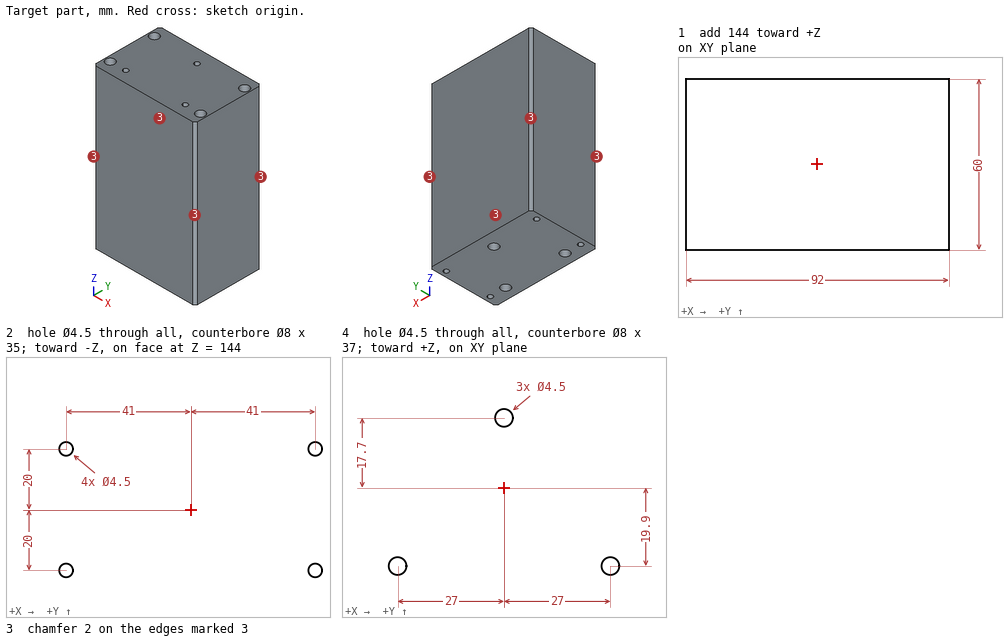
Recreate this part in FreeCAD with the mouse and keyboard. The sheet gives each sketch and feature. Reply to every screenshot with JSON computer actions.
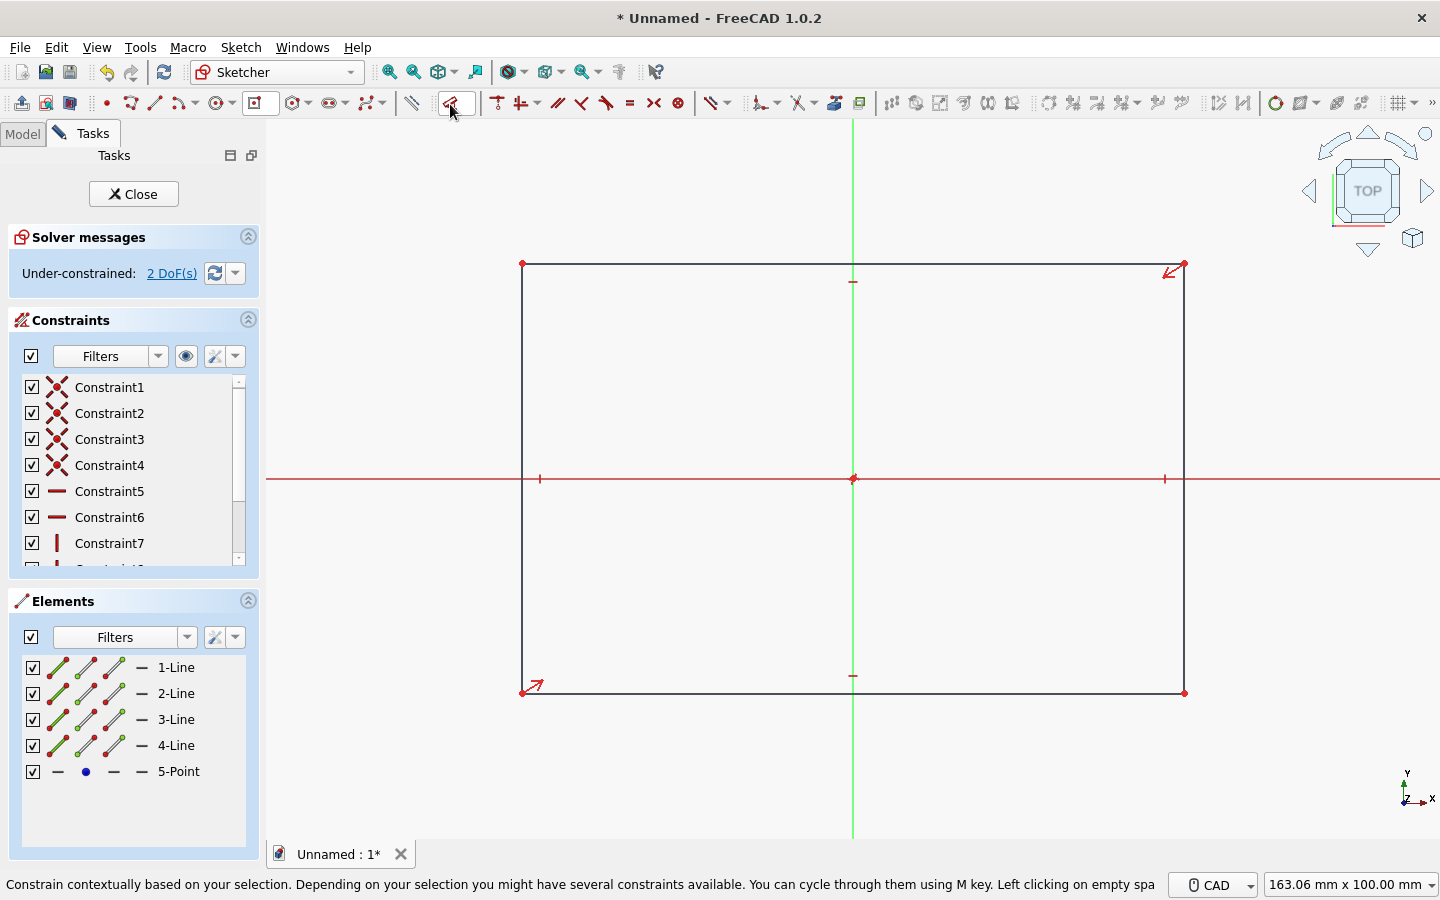
{"action": "left_click", "coordinate": [721, 694]}
{"action": "left_click", "coordinate": [701, 728]}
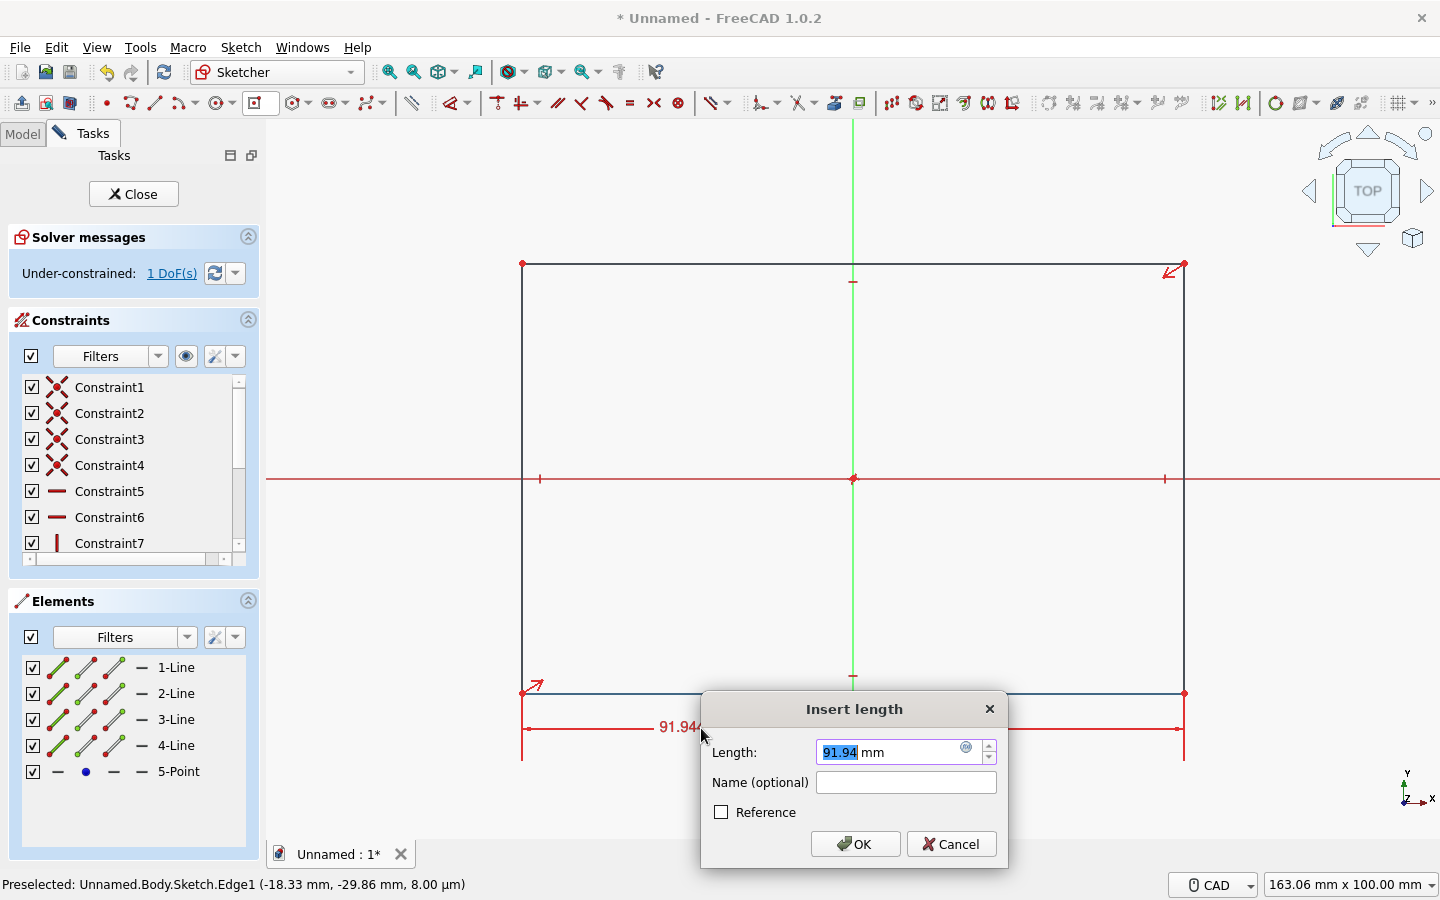
{"action": "type", "text": "92"}
{"action": "key", "text": "Return"}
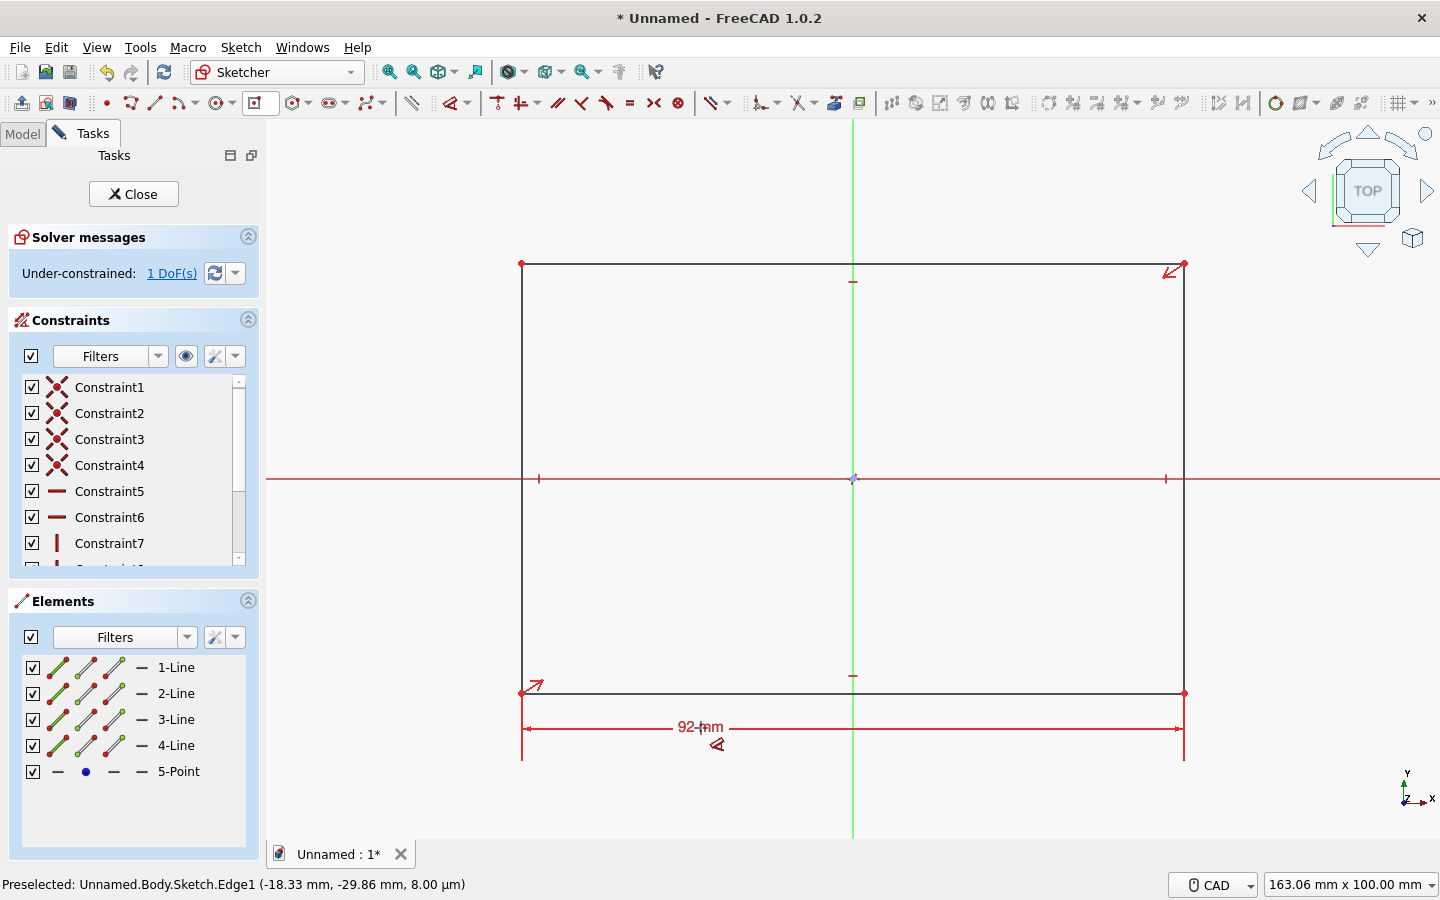
{"action": "left_click", "coordinate": [1184, 565]}
{"action": "left_click", "coordinate": [1218, 380]}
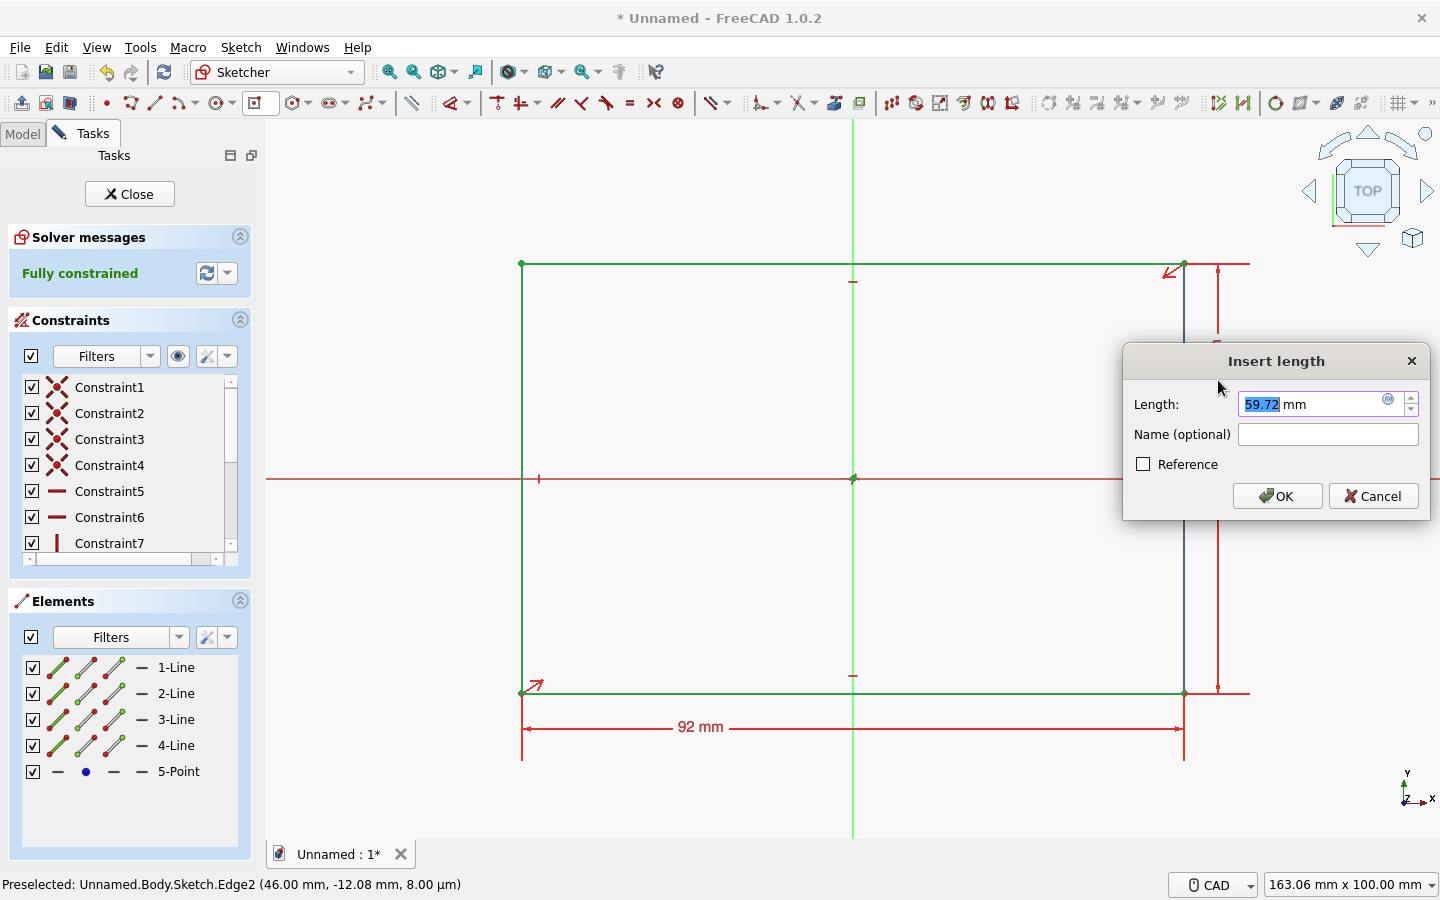
{"action": "type", "text": "60"}
{"action": "key", "text": "Return"}
{"action": "key", "text": "Escape"}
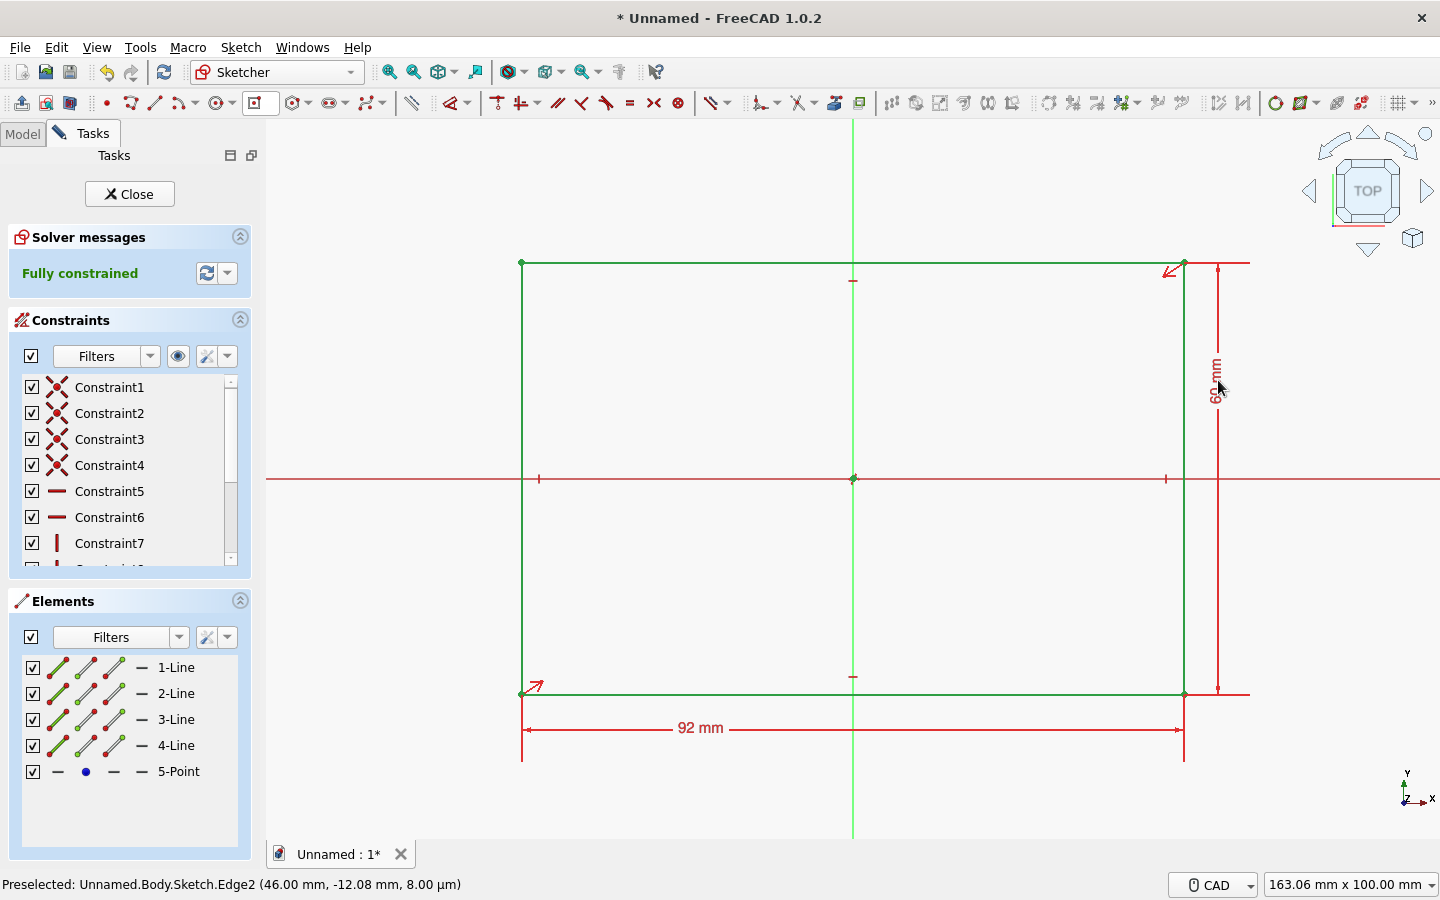
{"action": "left_click", "coordinate": [130, 194]}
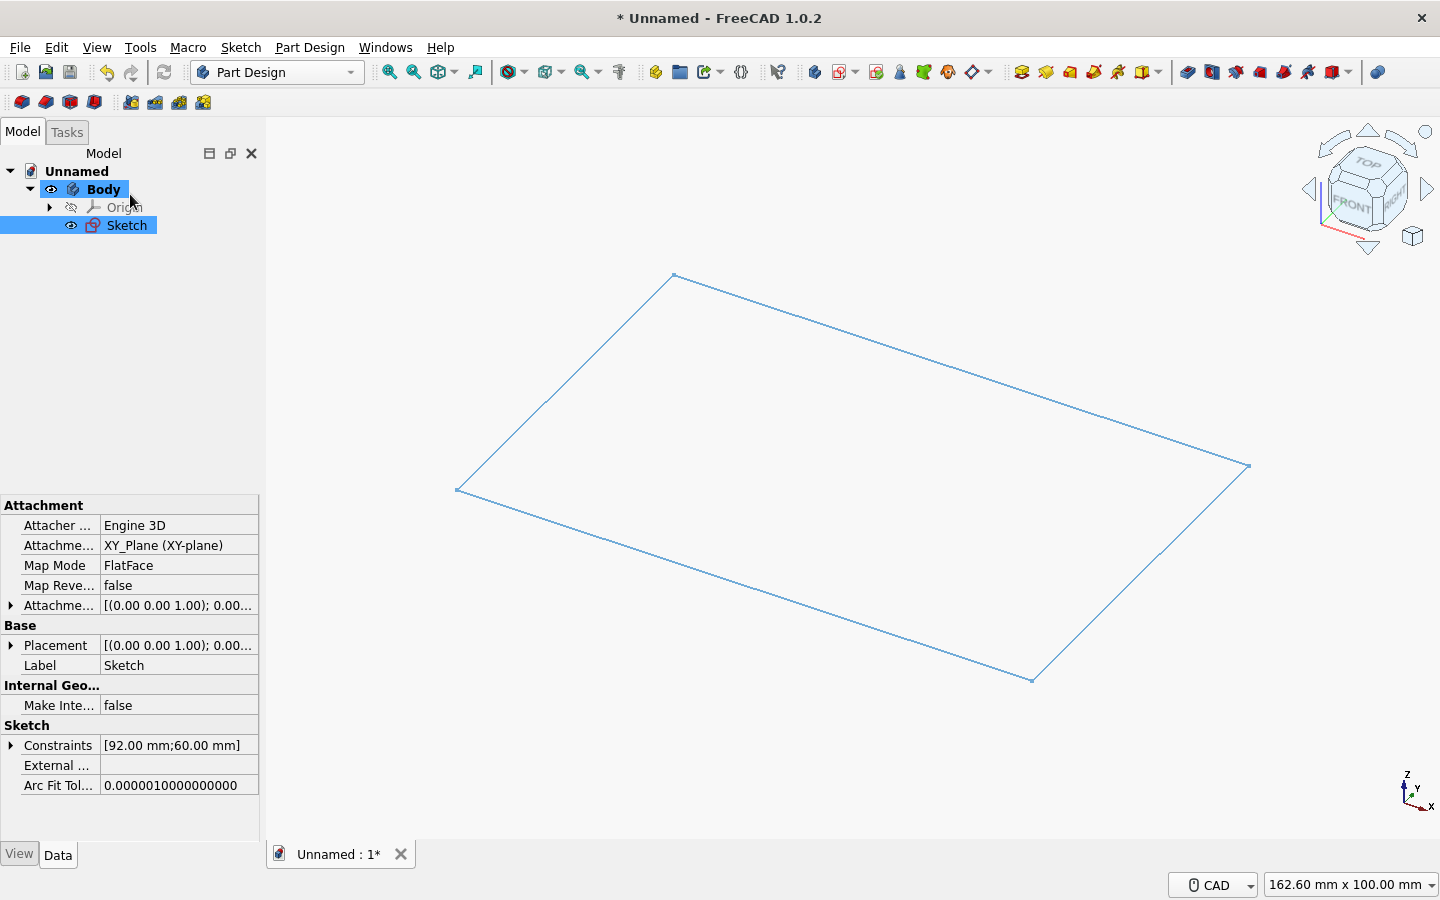
{"action": "left_click", "coordinate": [1022, 72]}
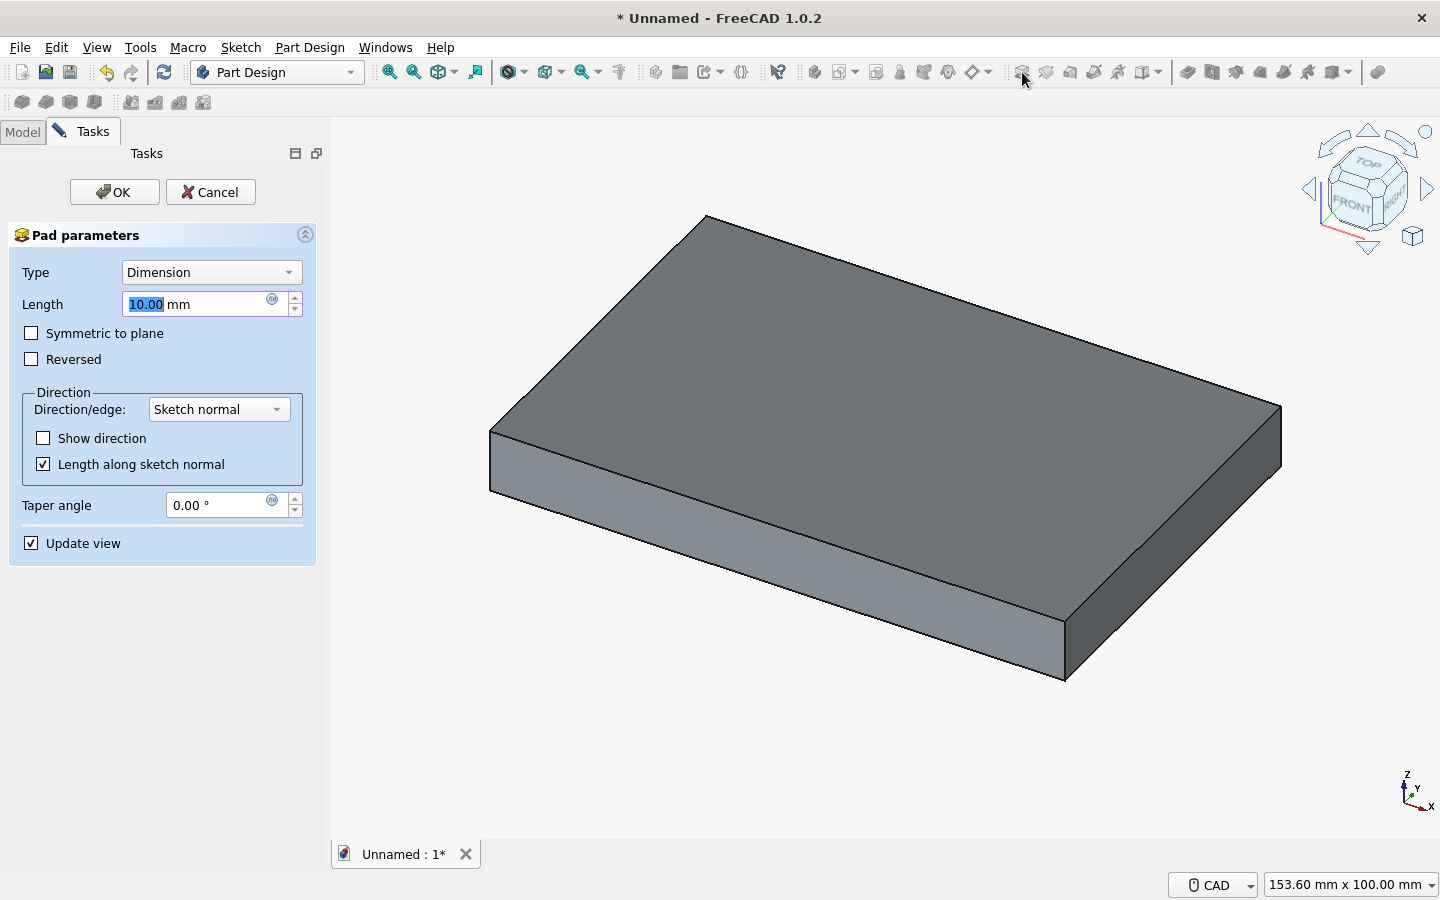
{"action": "type", "text": "144"}
{"action": "key", "text": "Tab"}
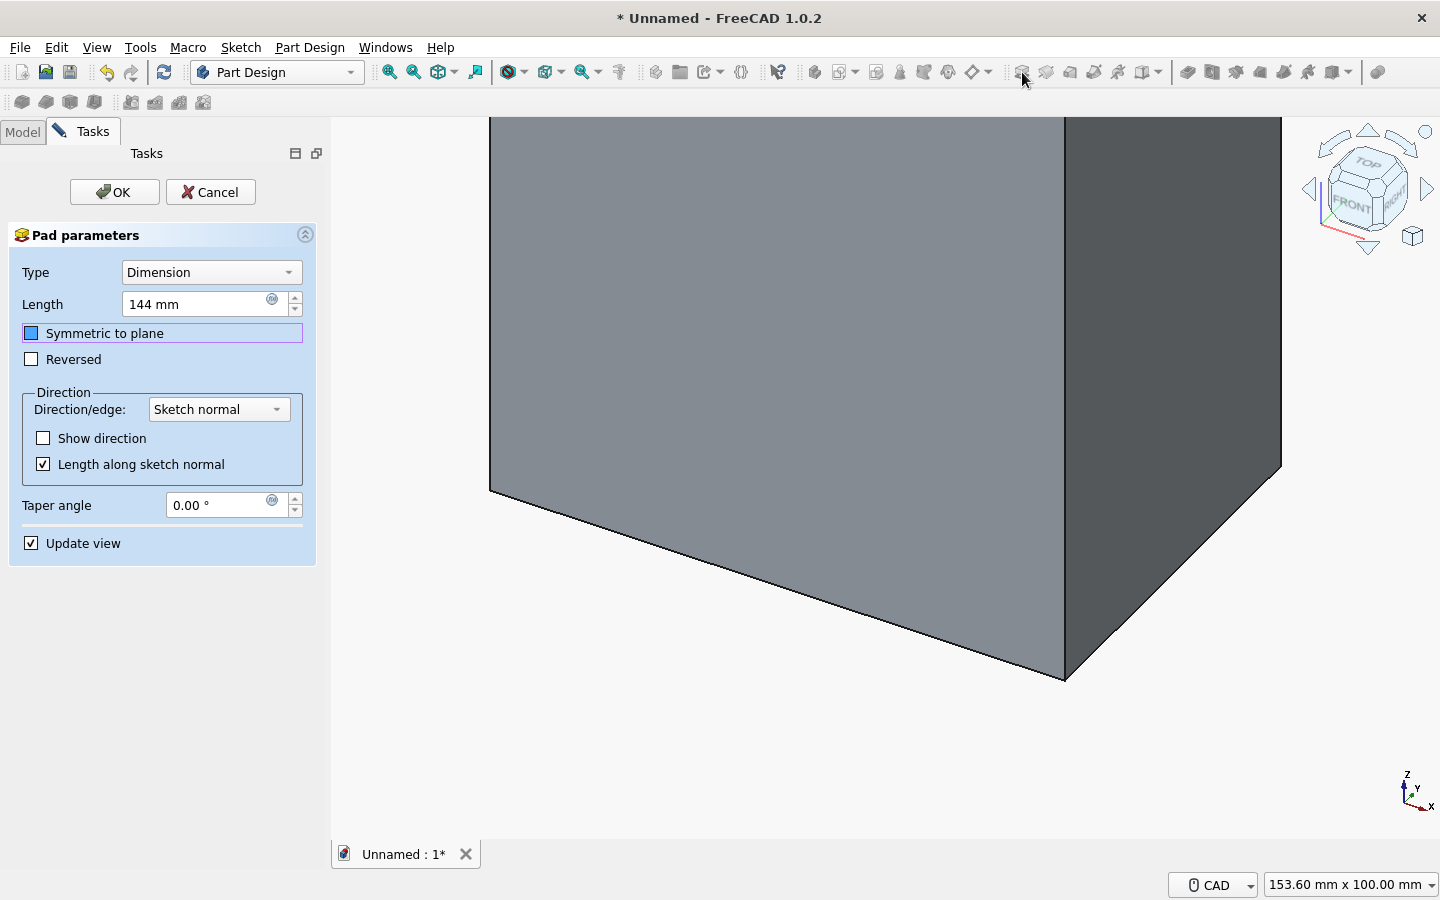
{"action": "left_click", "coordinate": [115, 192]}